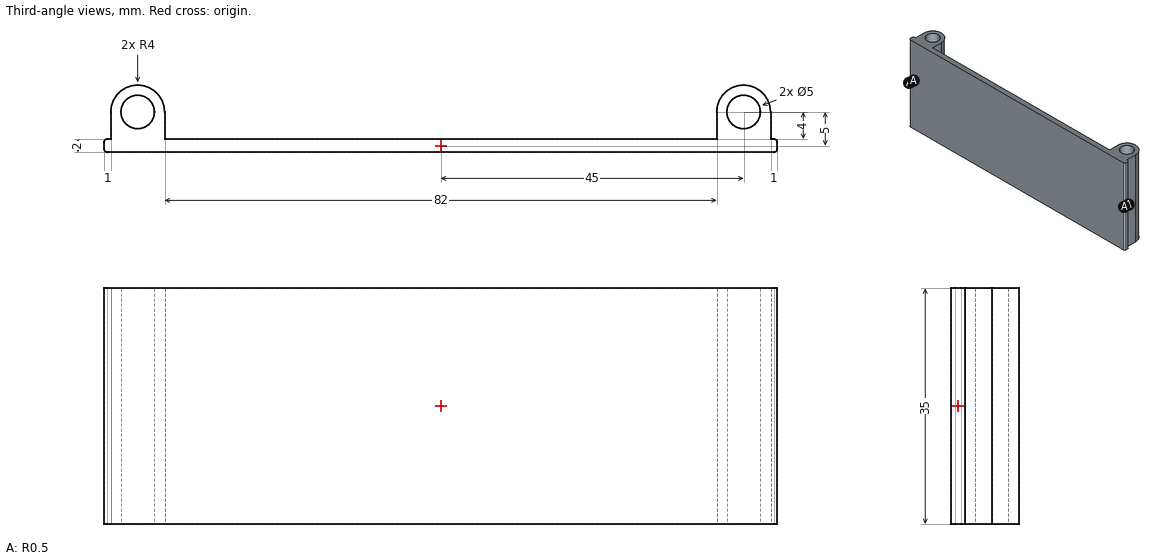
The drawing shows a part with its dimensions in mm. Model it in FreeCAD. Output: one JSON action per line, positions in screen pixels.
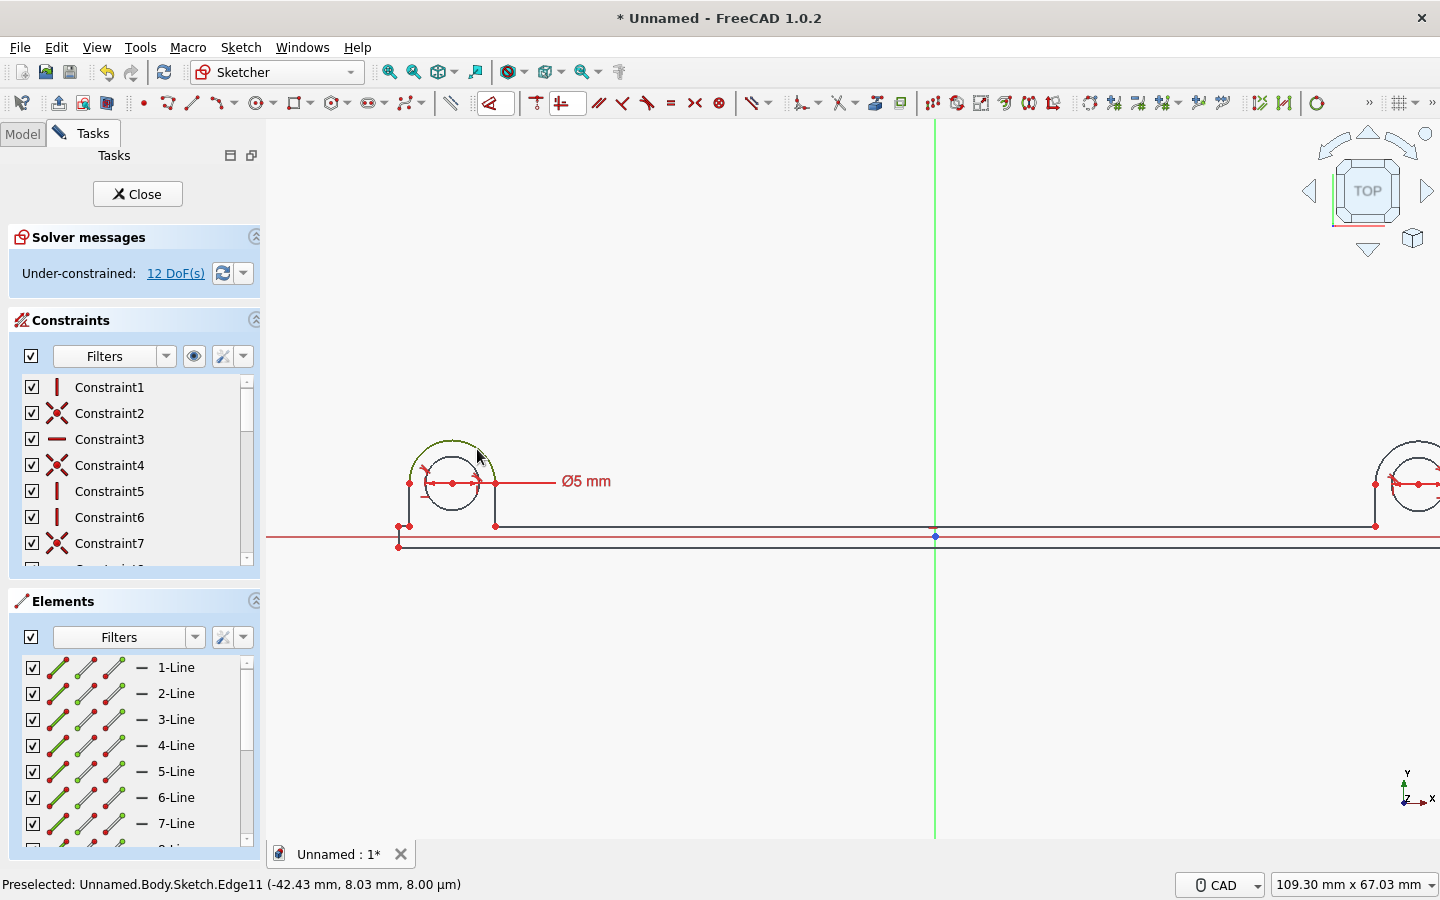
{"action": "scroll", "coordinate": [478, 449], "scroll_direction": "down", "scroll_amount": 2}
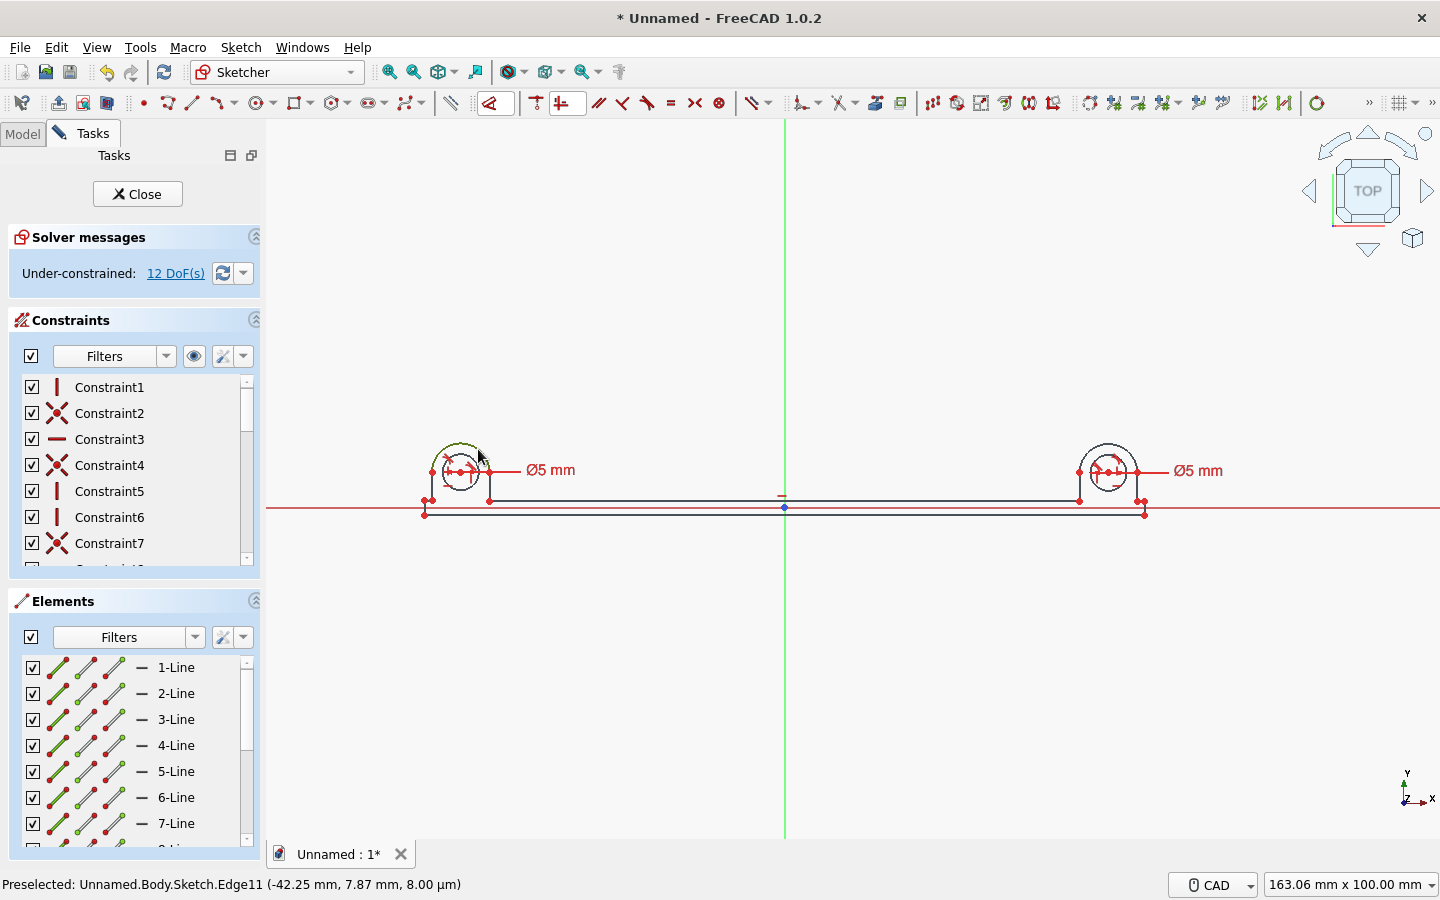
{"action": "scroll", "coordinate": [1125, 450], "scroll_direction": "up", "scroll_amount": 2}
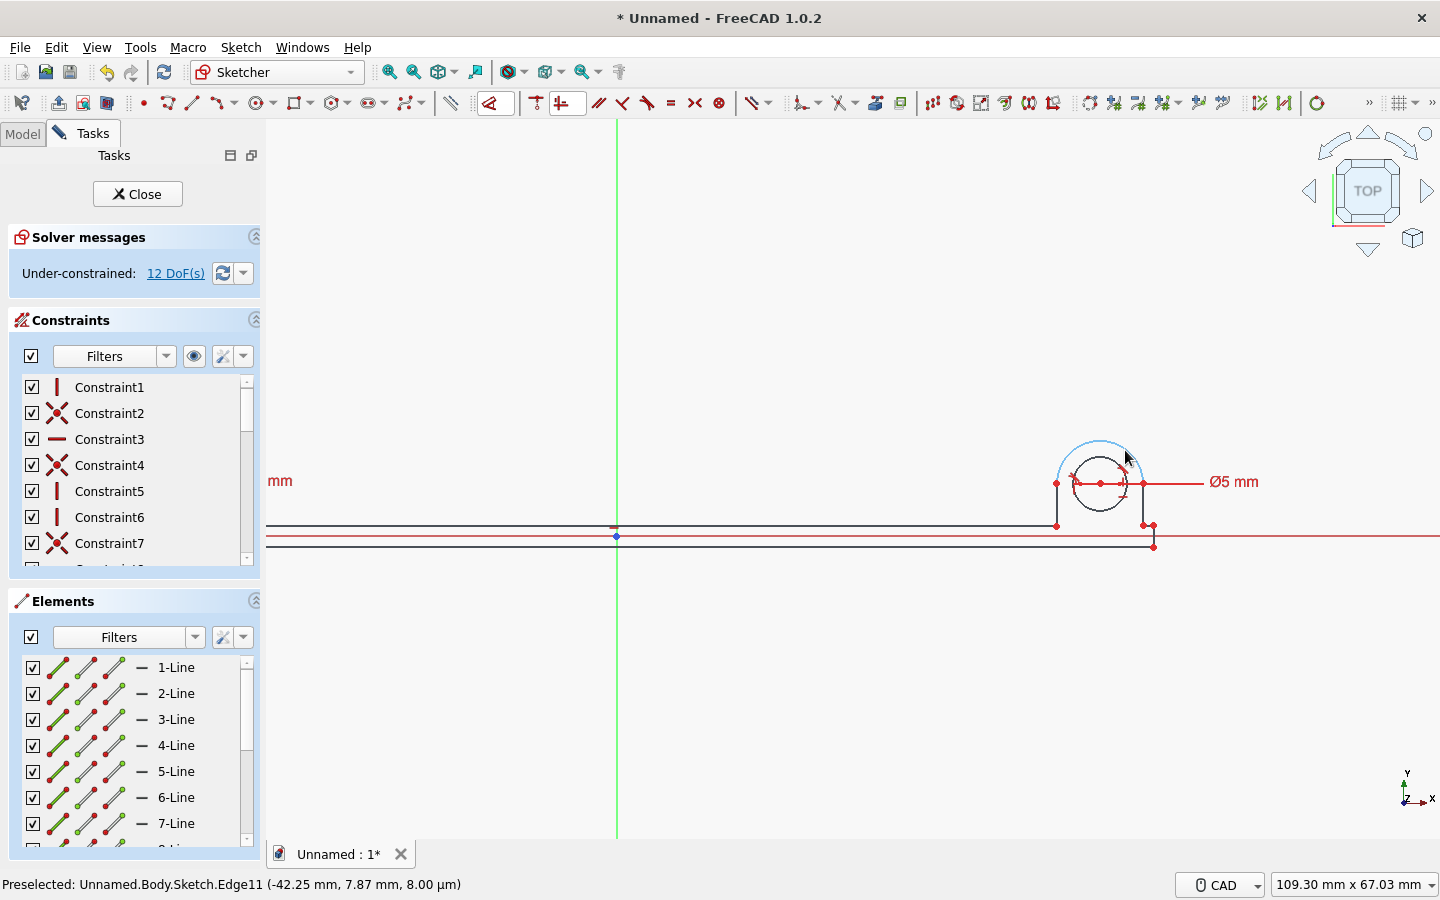
{"action": "left_click", "coordinate": [1125, 449]}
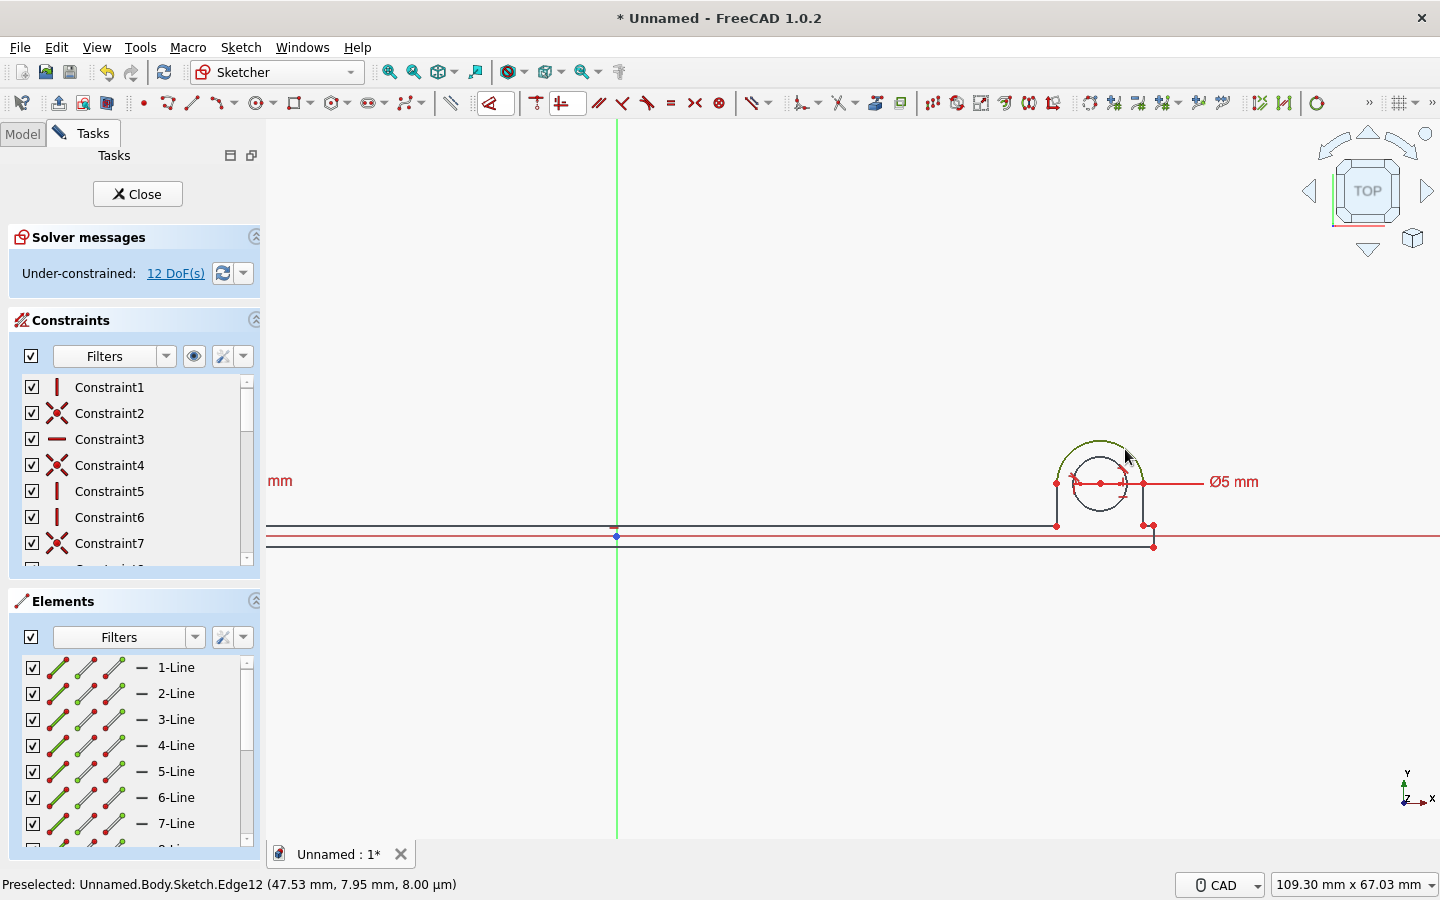
{"action": "left_click", "coordinate": [672, 104]}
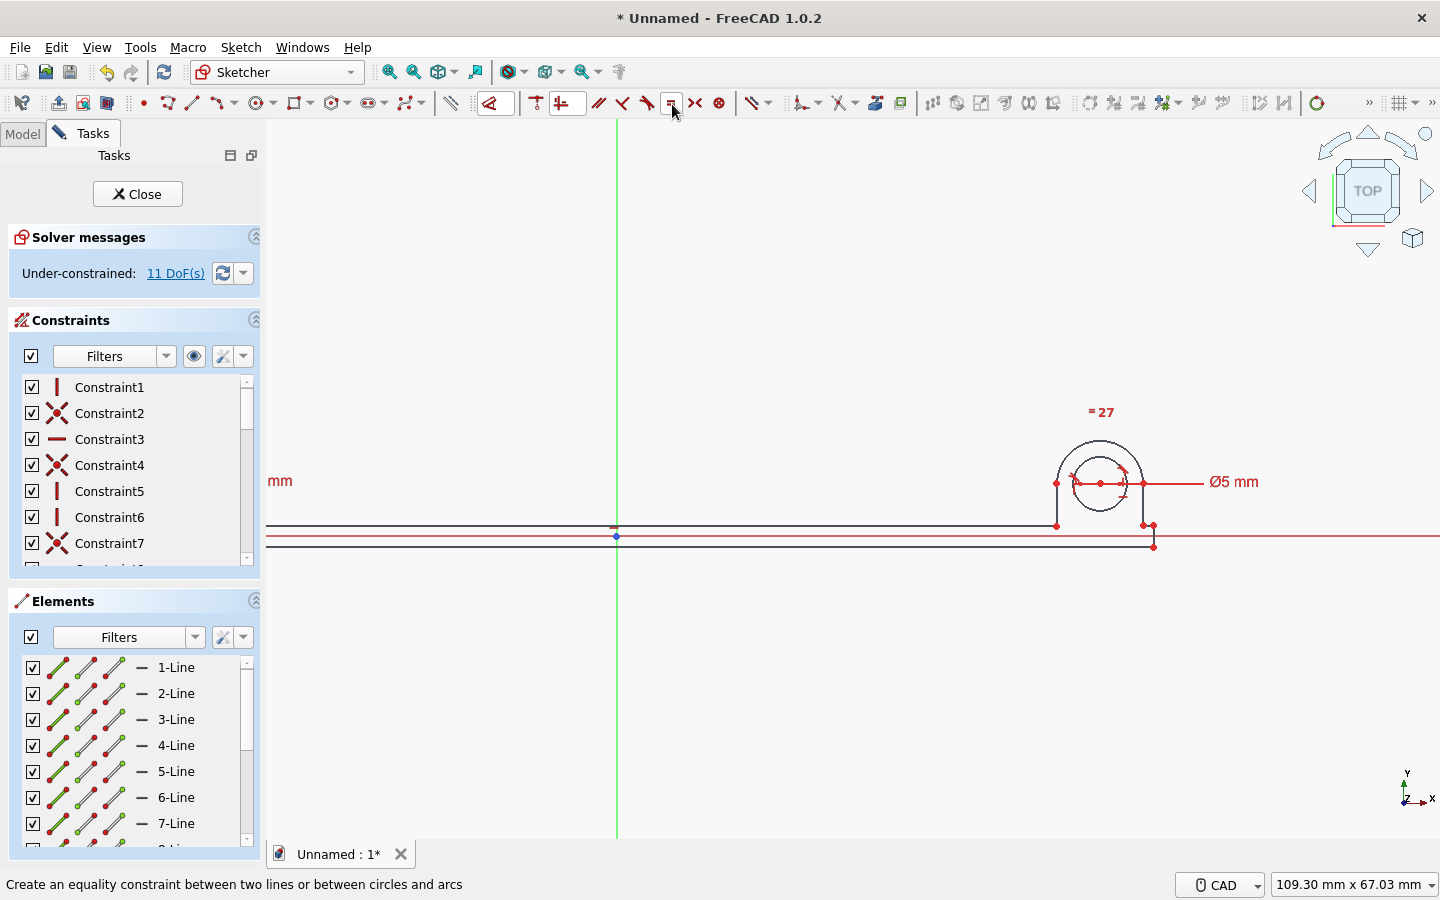
{"action": "left_click", "coordinate": [490, 104]}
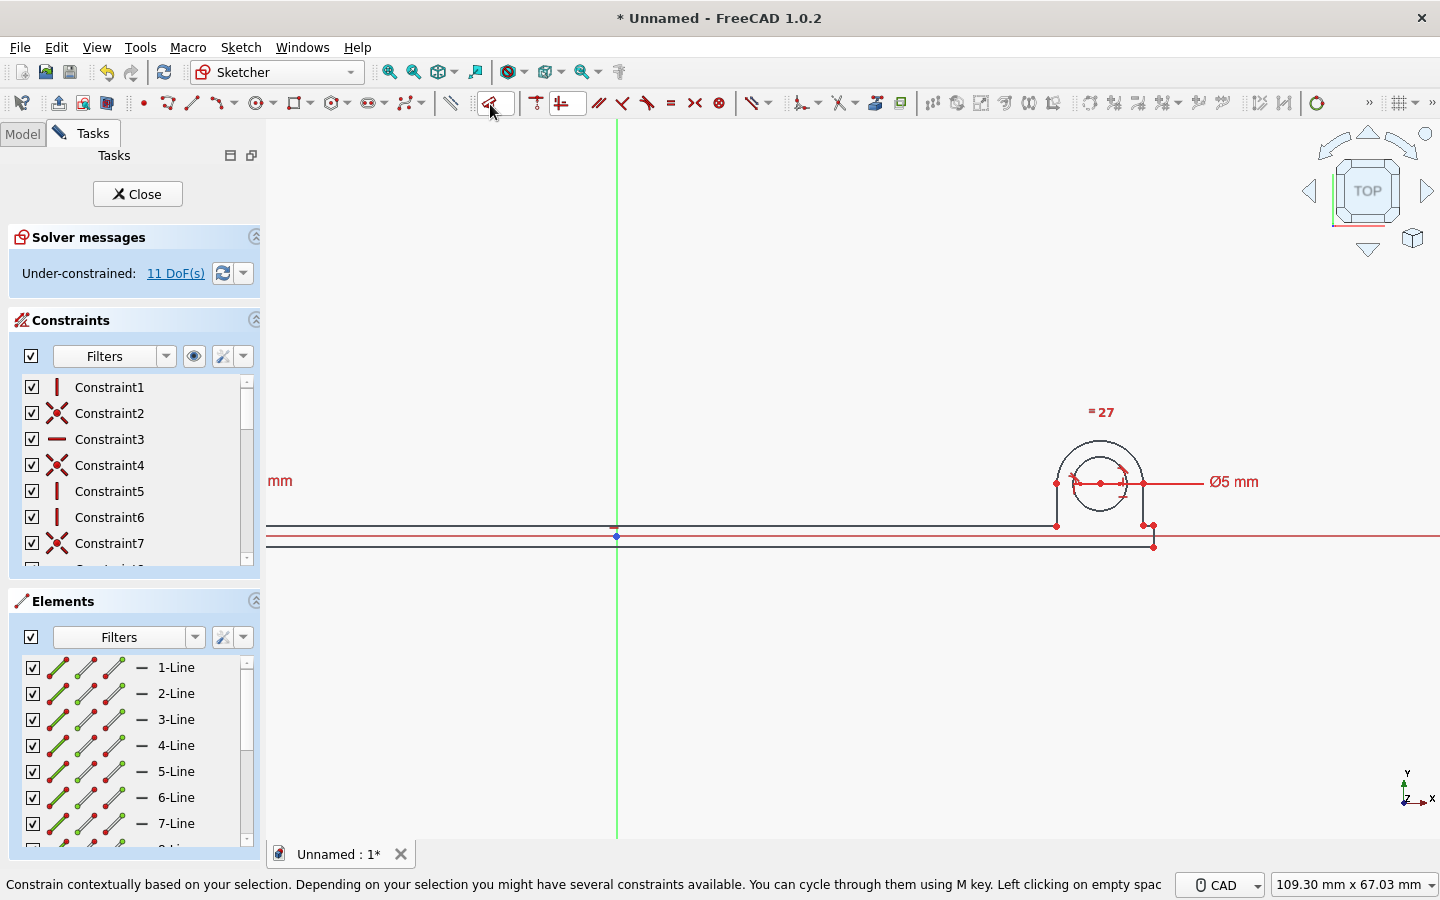
{"action": "scroll", "coordinate": [1125, 450], "scroll_direction": "down", "scroll_amount": 2}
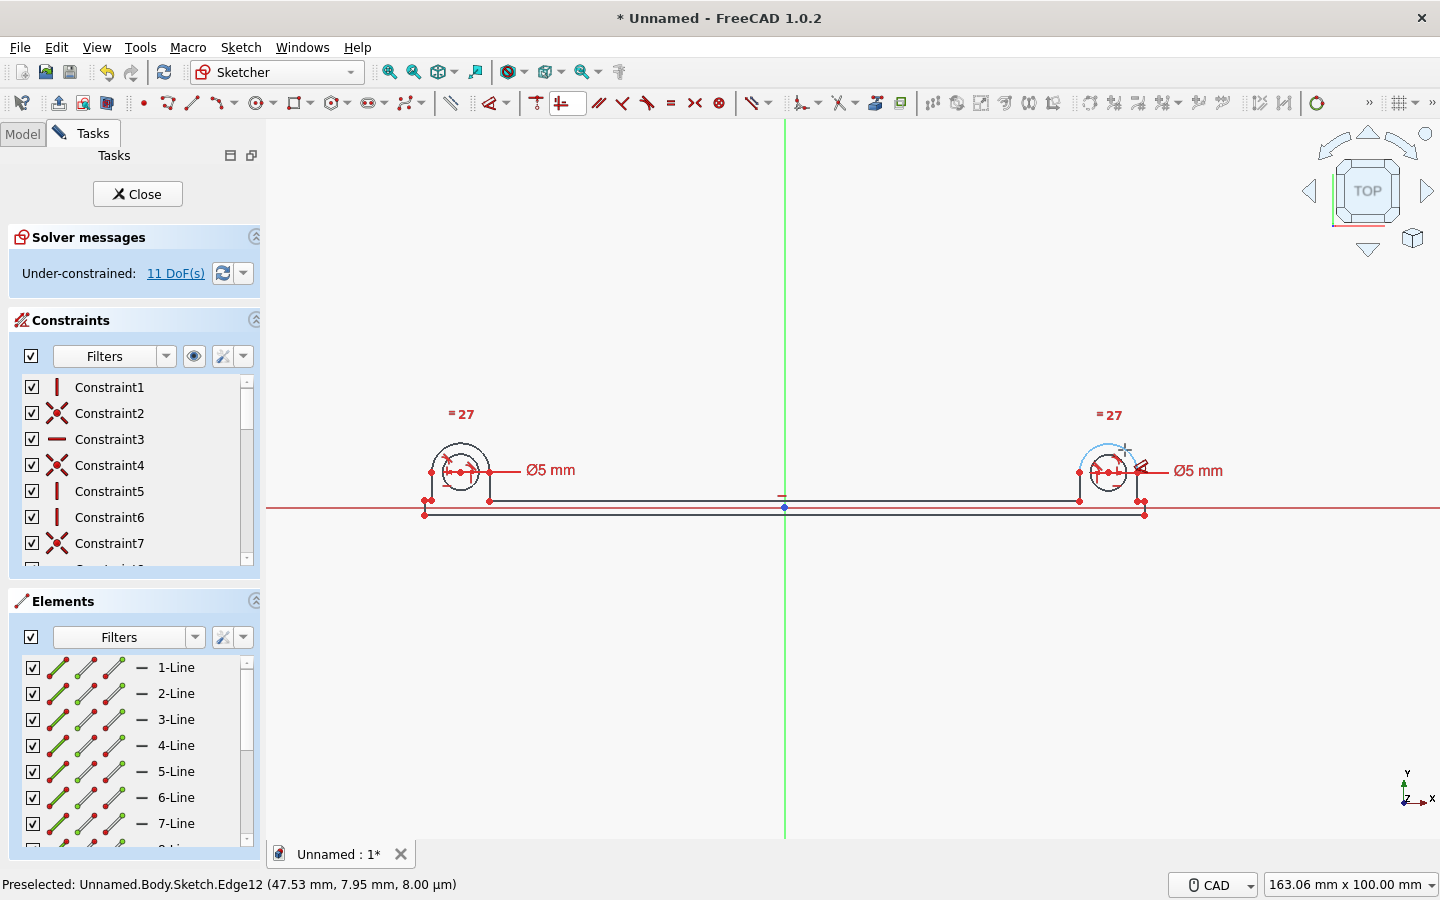
{"action": "scroll", "coordinate": [478, 449], "scroll_direction": "up", "scroll_amount": 2}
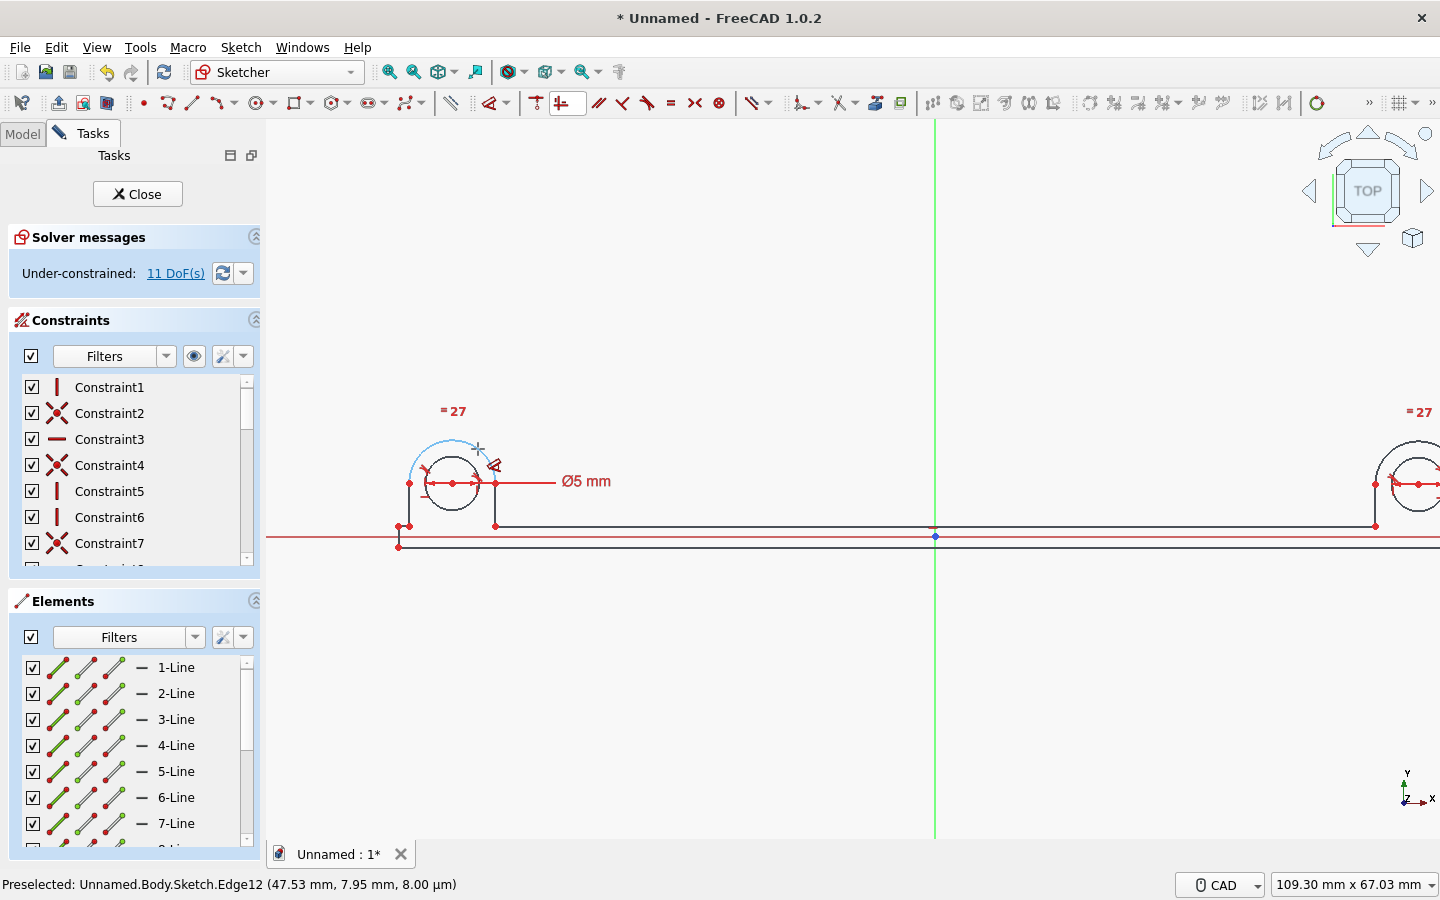
{"action": "left_click", "coordinate": [478, 449]}
{"action": "left_click", "coordinate": [497, 423]}